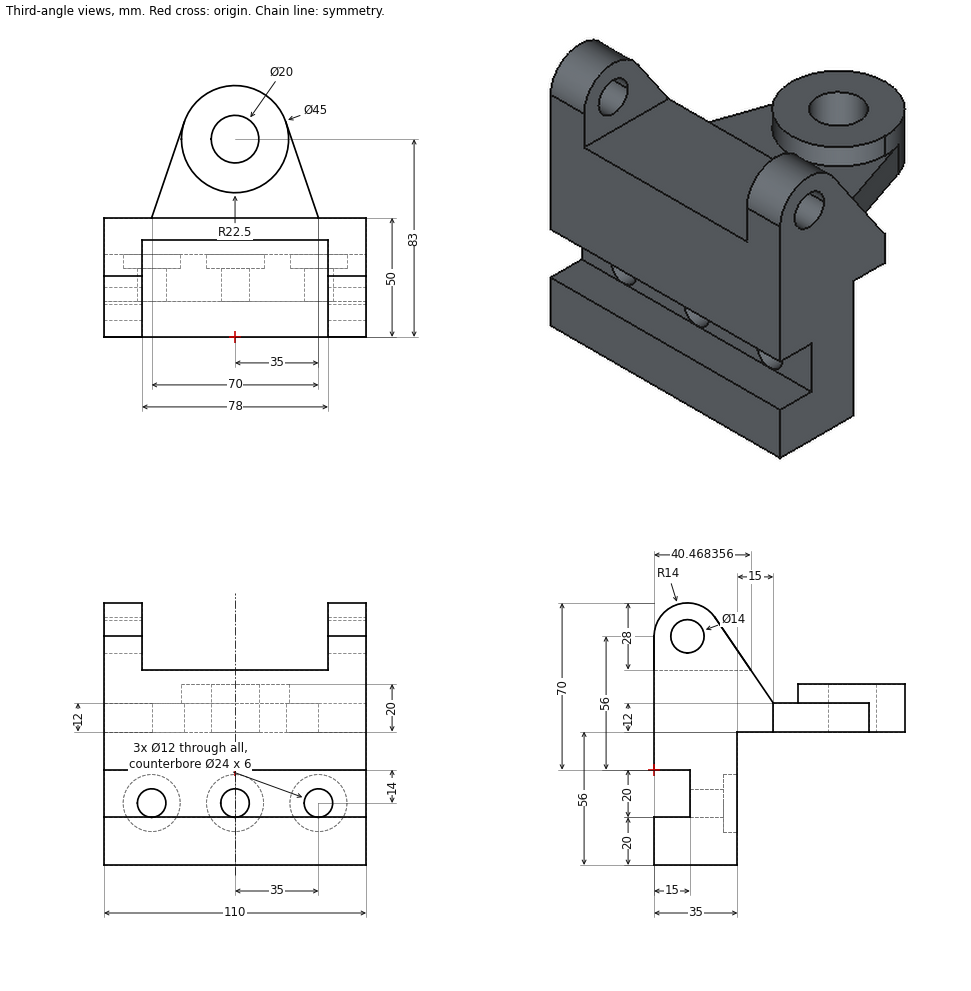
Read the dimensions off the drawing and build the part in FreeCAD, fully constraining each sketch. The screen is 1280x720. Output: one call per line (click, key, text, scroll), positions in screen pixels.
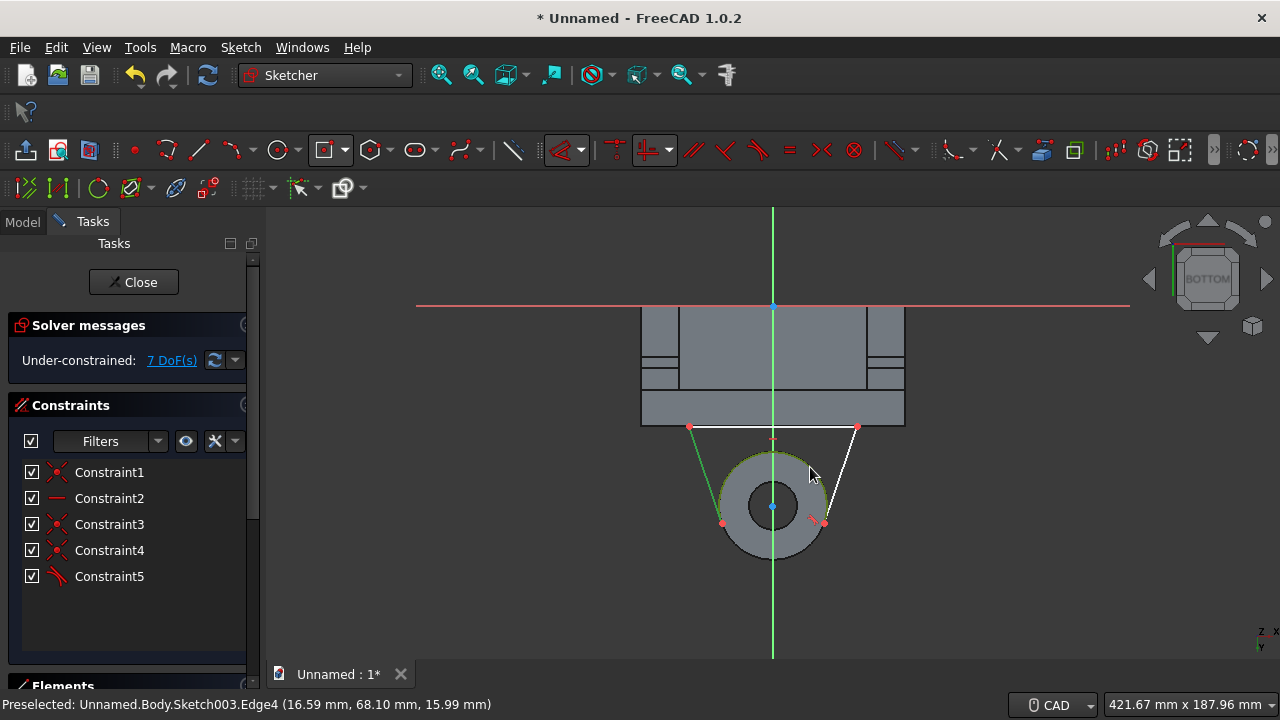
click(758, 150)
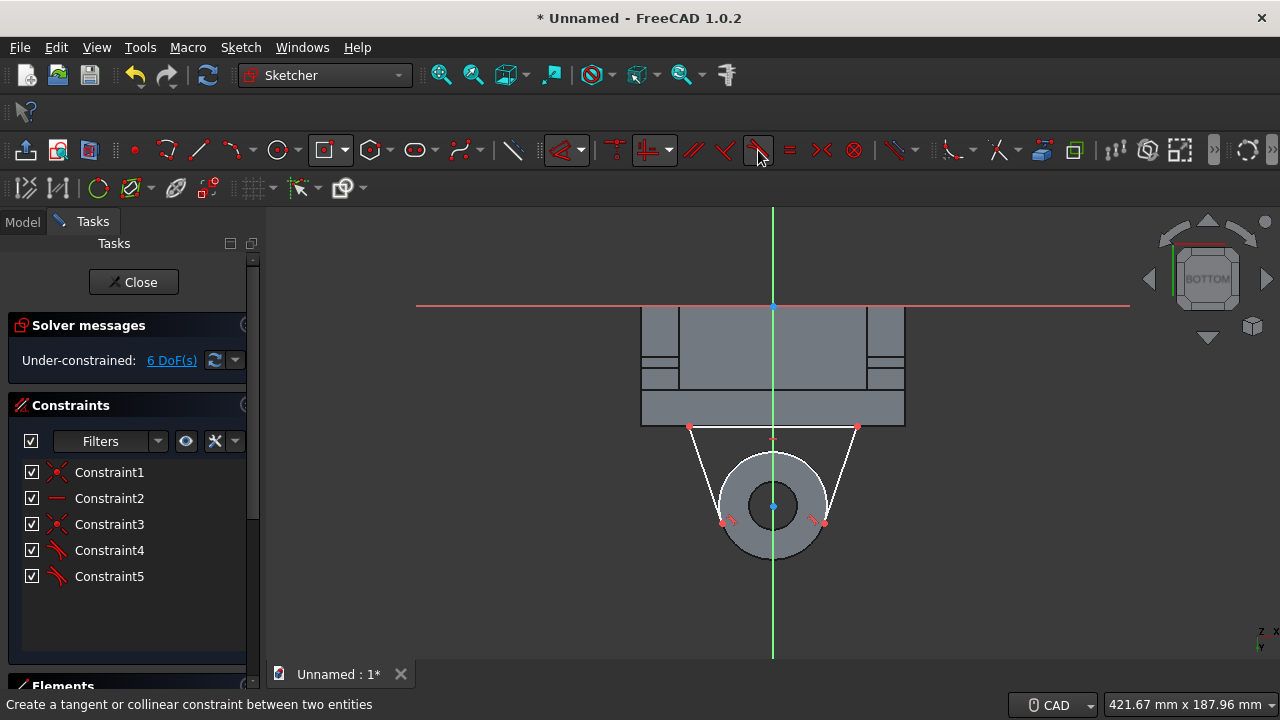
click(773, 506)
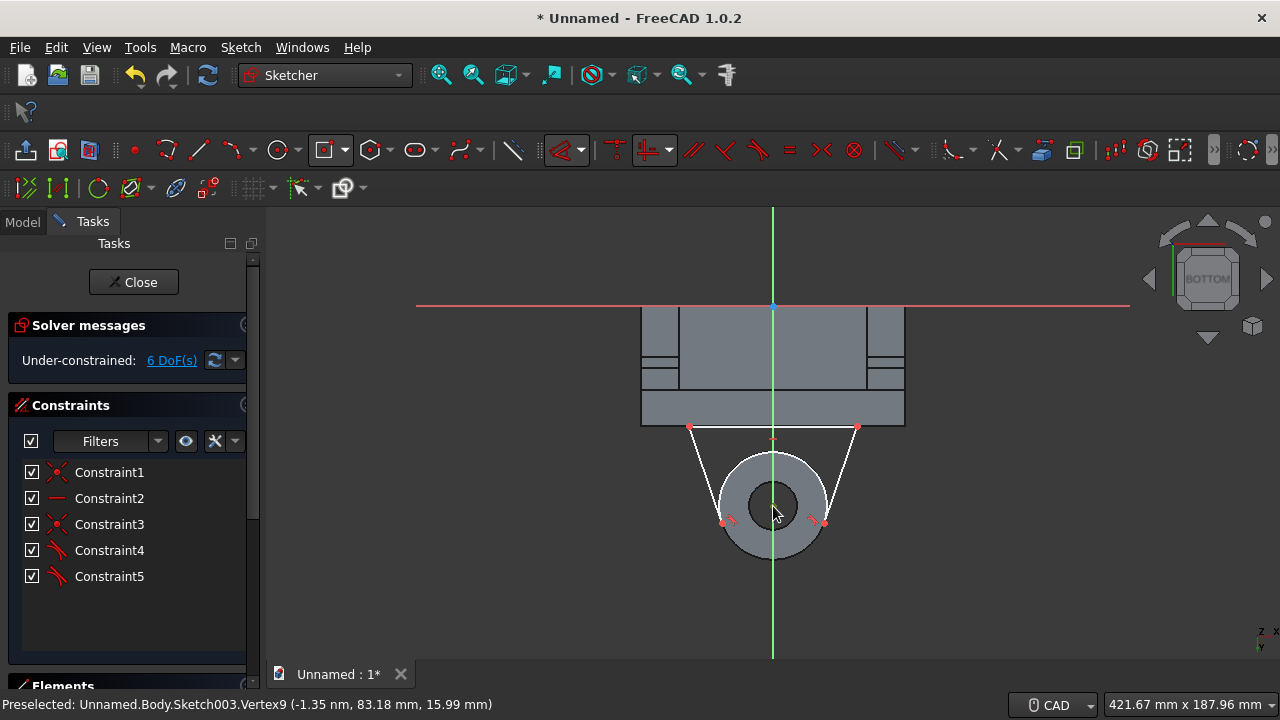
click(773, 603)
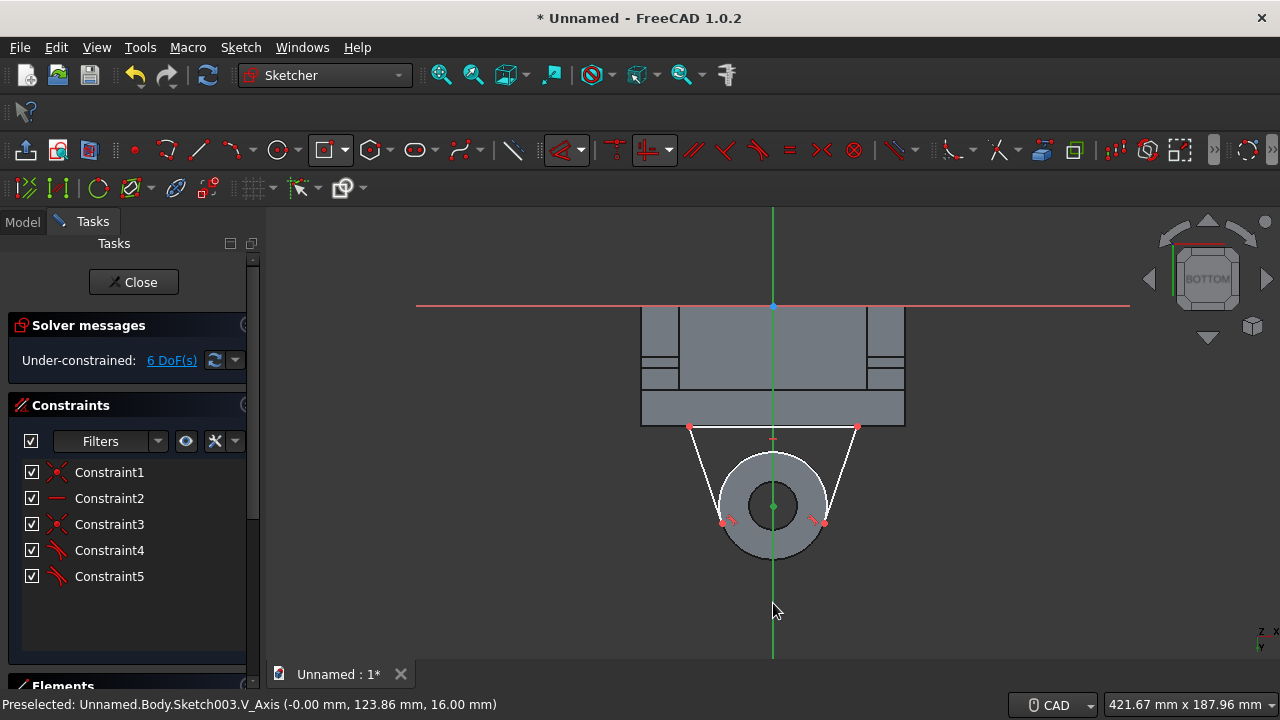
click(616, 150)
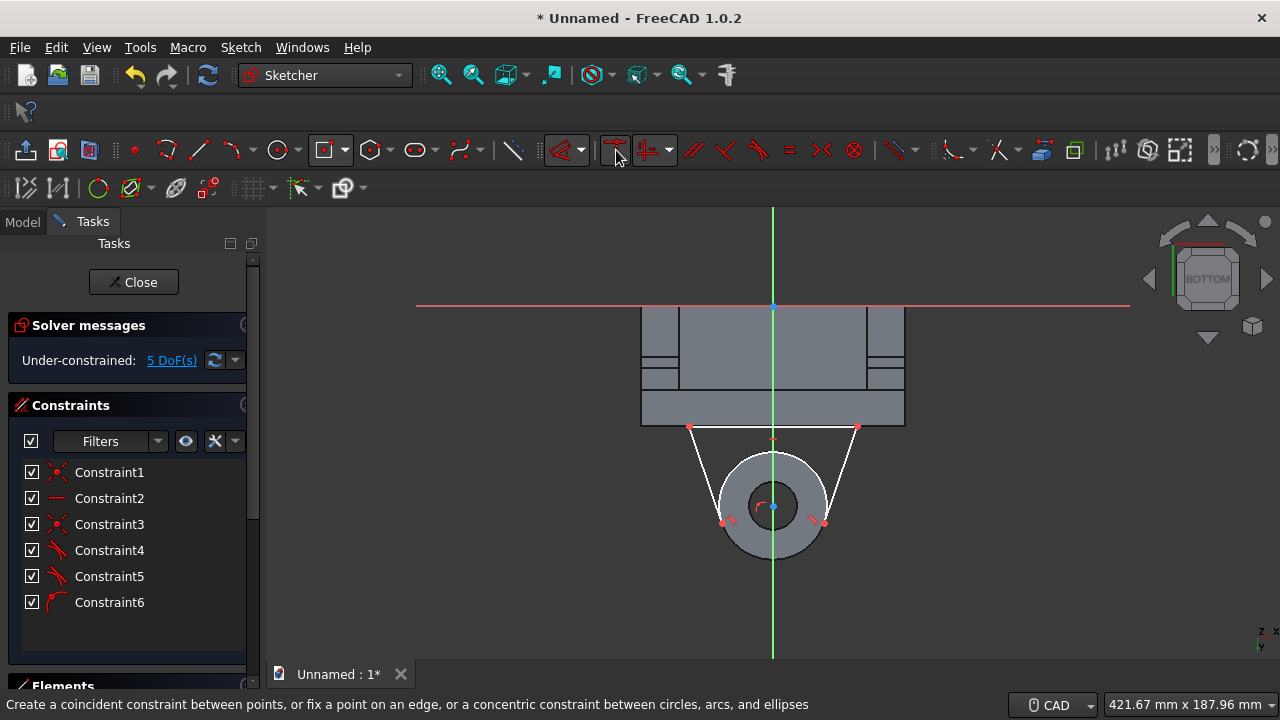
click(810, 467)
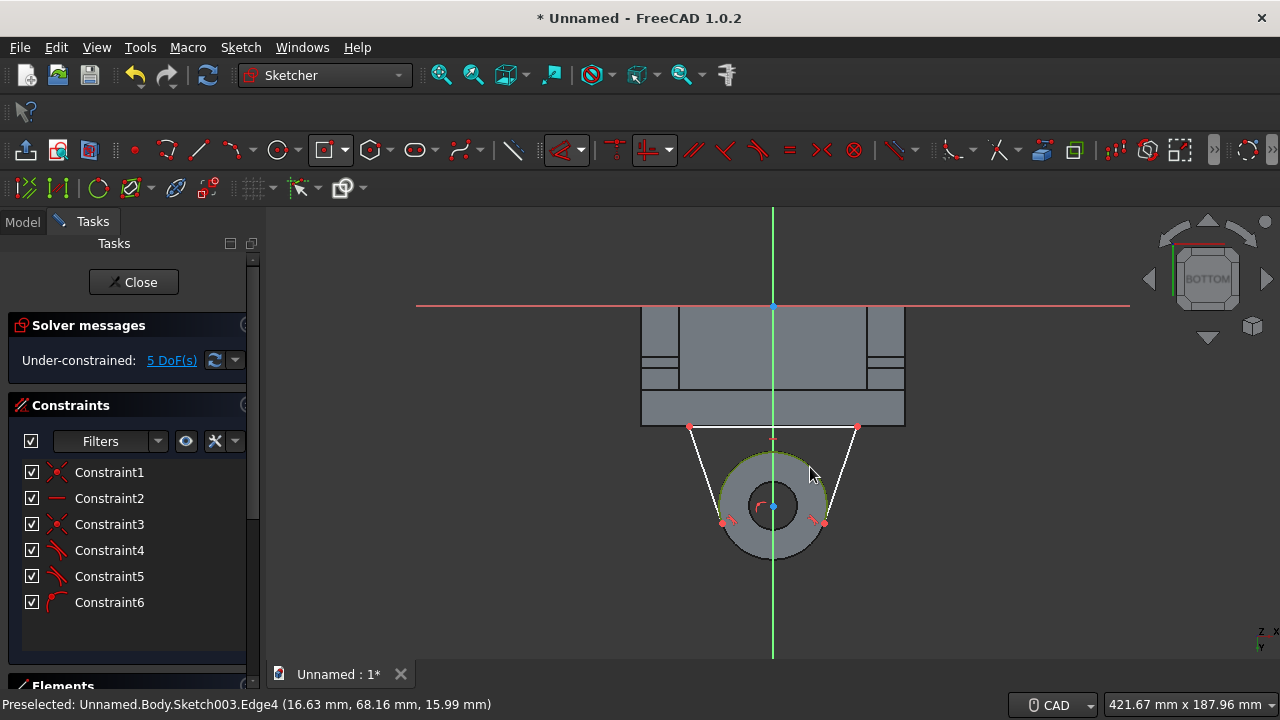
key(k)
key(r)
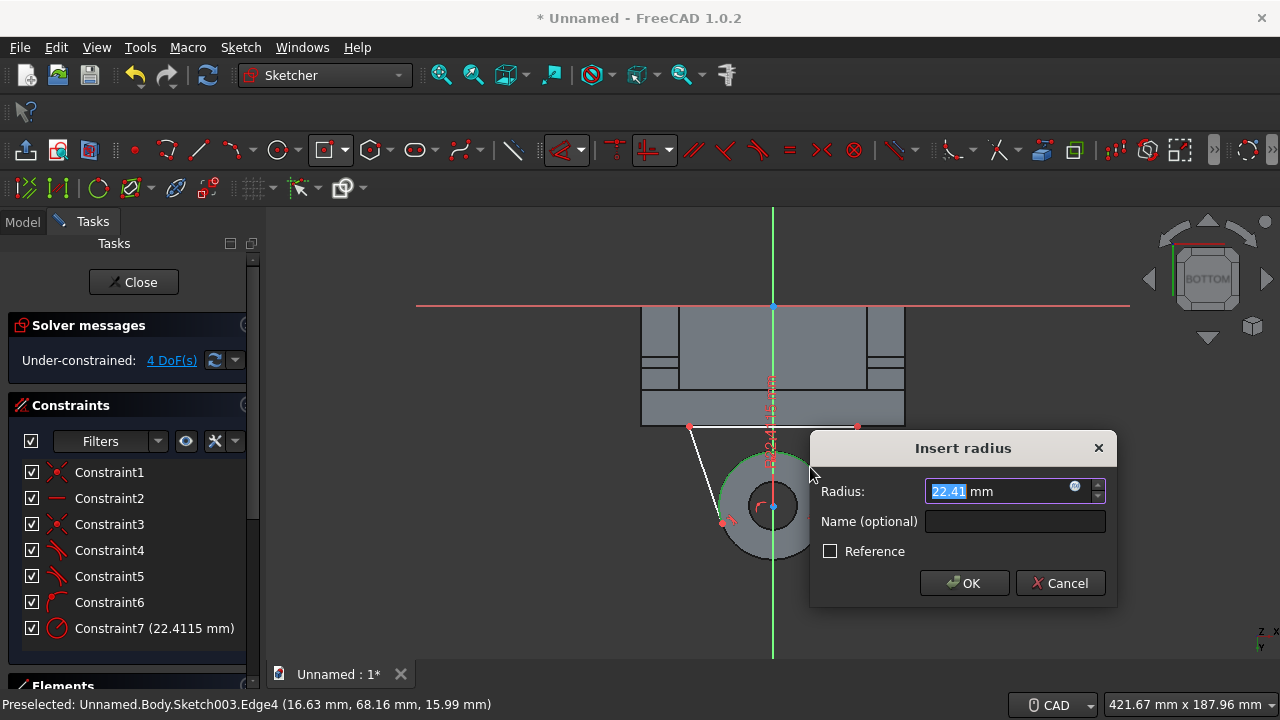
text(22.5)
key(Return)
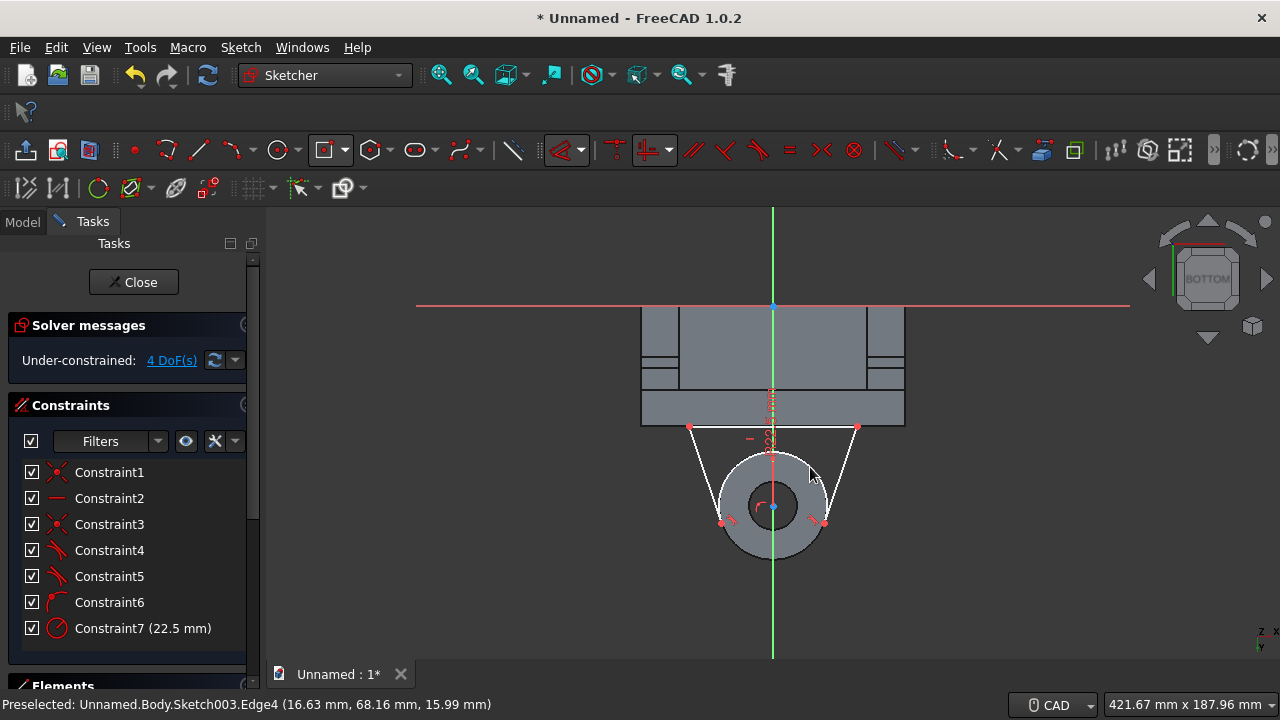
click(807, 427)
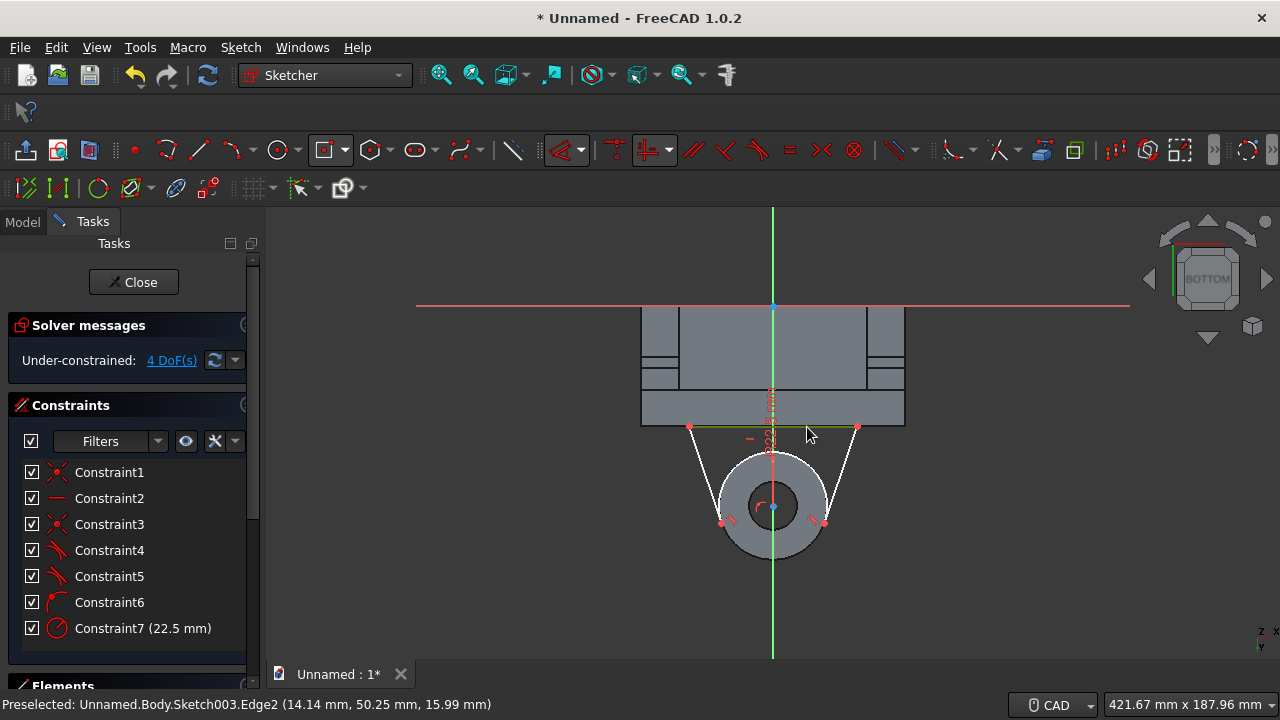
key(l)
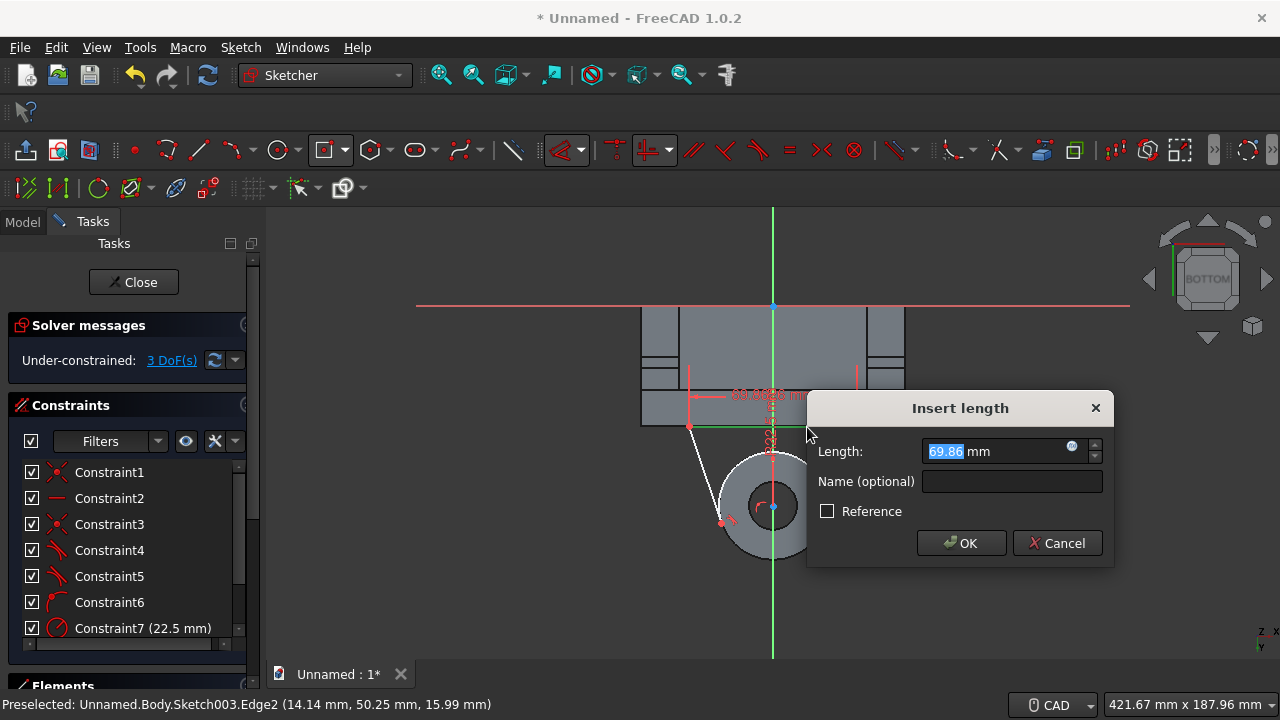
text(70)
key(Return)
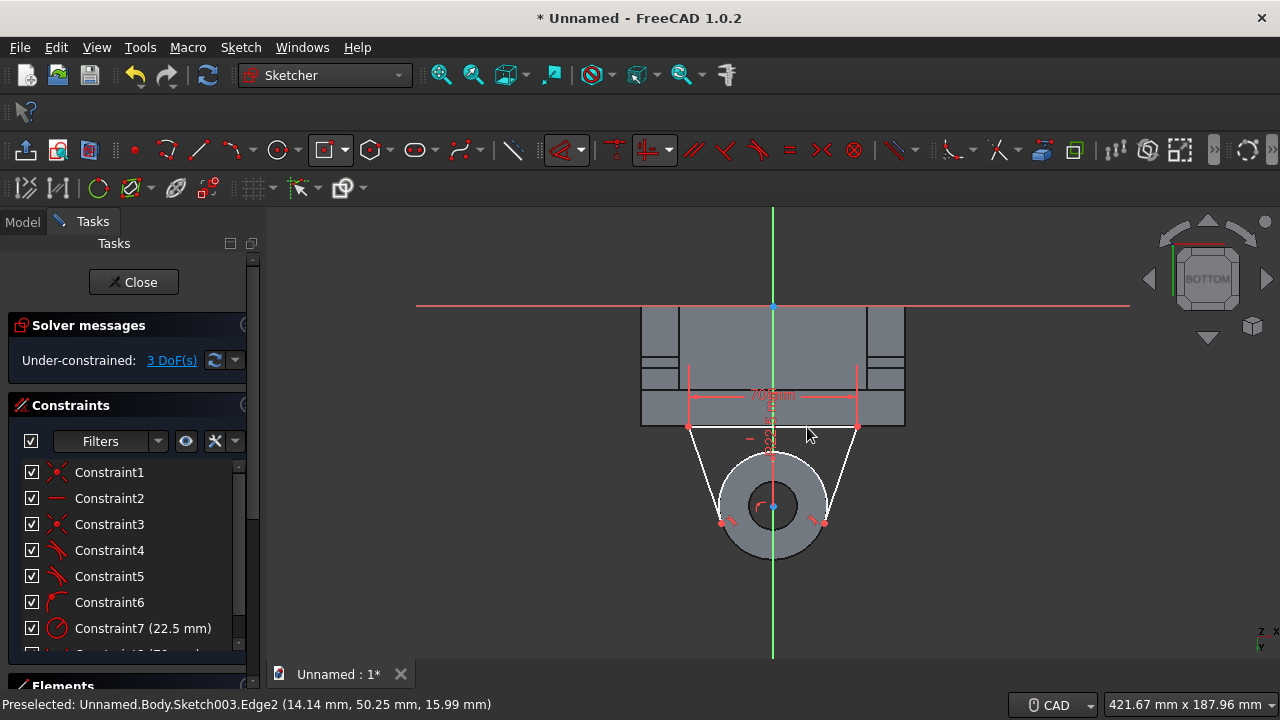
click(857, 427)